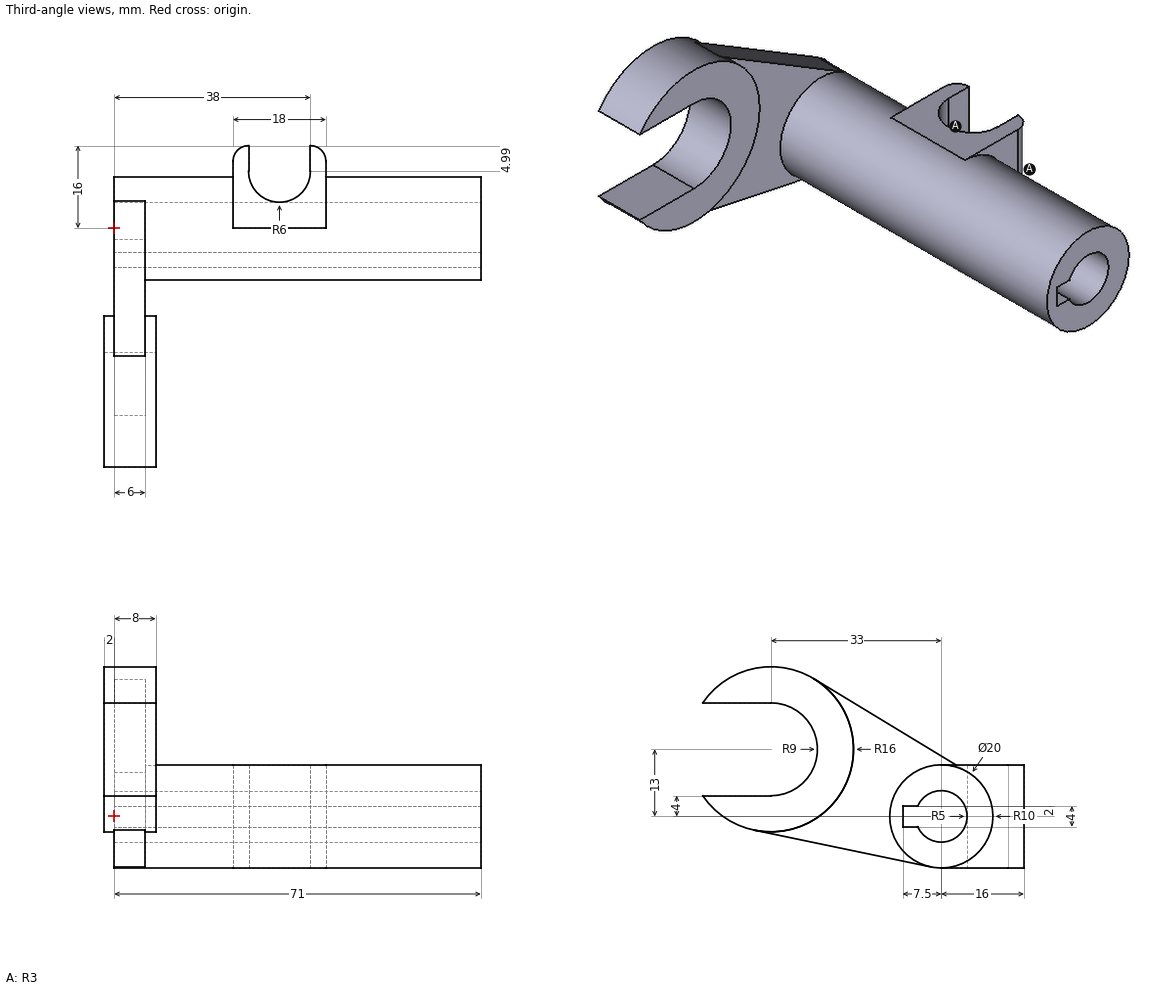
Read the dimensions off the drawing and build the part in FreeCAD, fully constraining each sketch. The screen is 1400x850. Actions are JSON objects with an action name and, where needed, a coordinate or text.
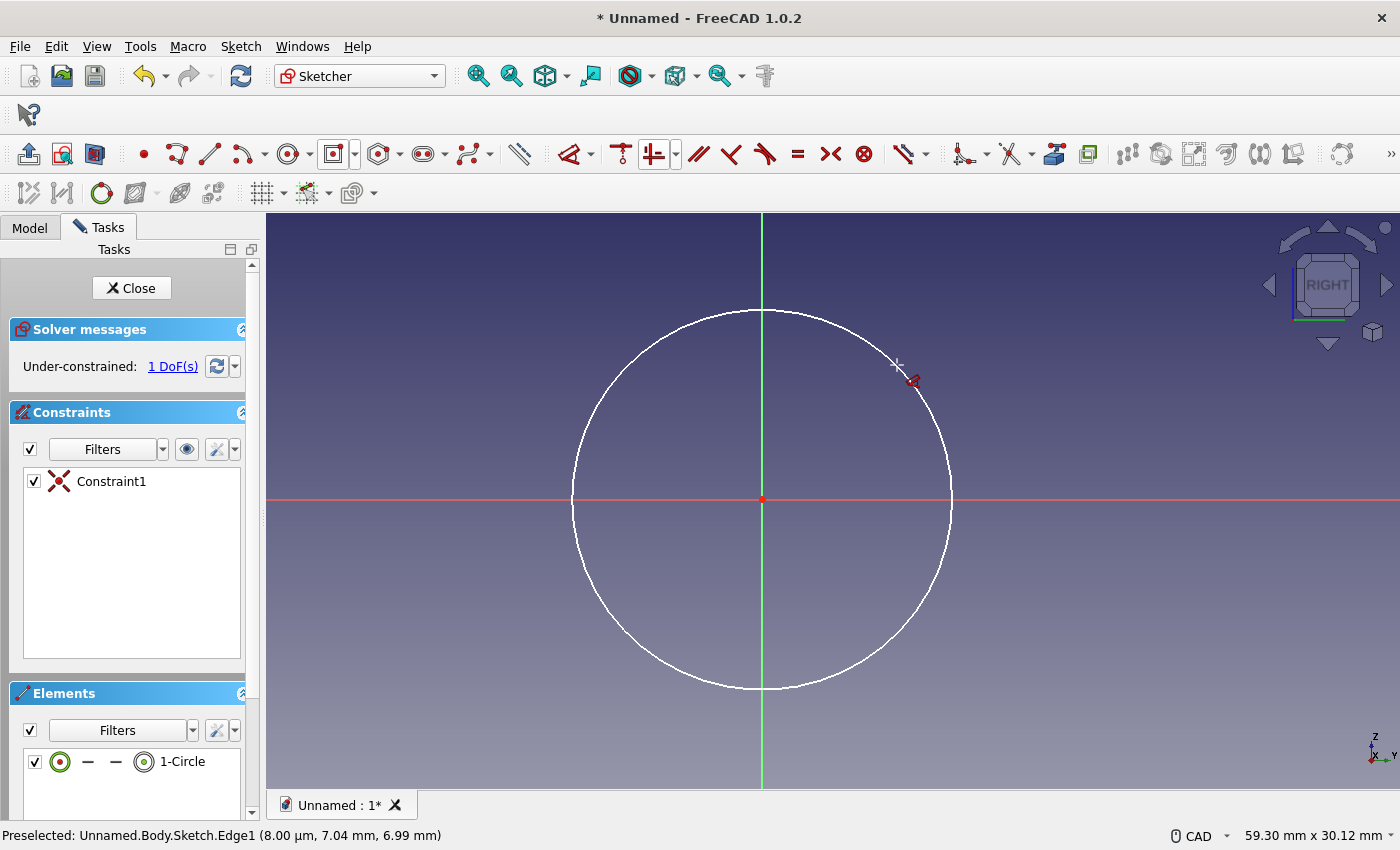
{"action": "left_click", "coordinate": [896, 365]}
{"action": "left_click", "coordinate": [919, 342]}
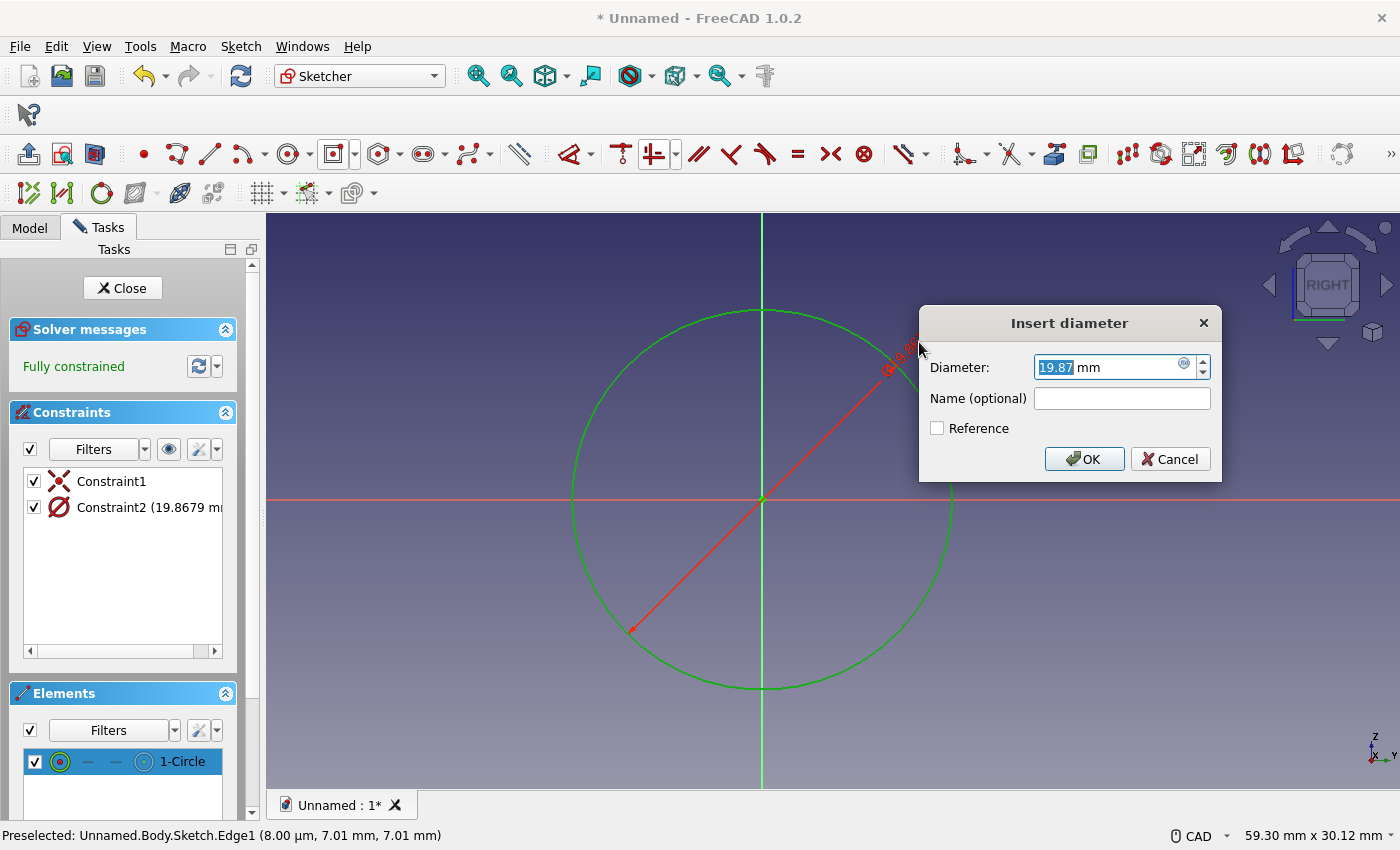
{"action": "type", "text": "20"}
{"action": "key", "text": "Return"}
{"action": "key", "text": "Escape"}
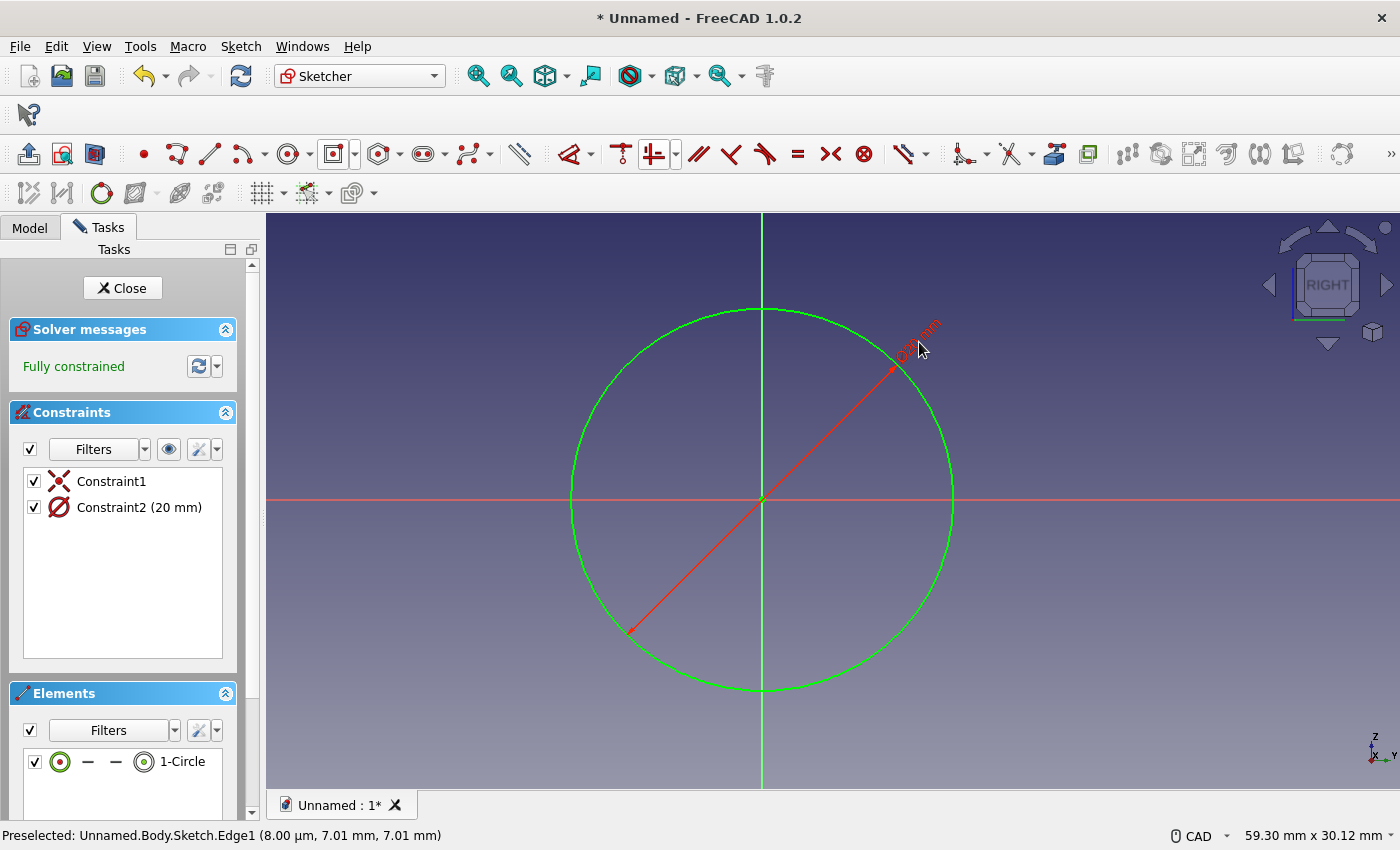
{"action": "left_click", "coordinate": [123, 288]}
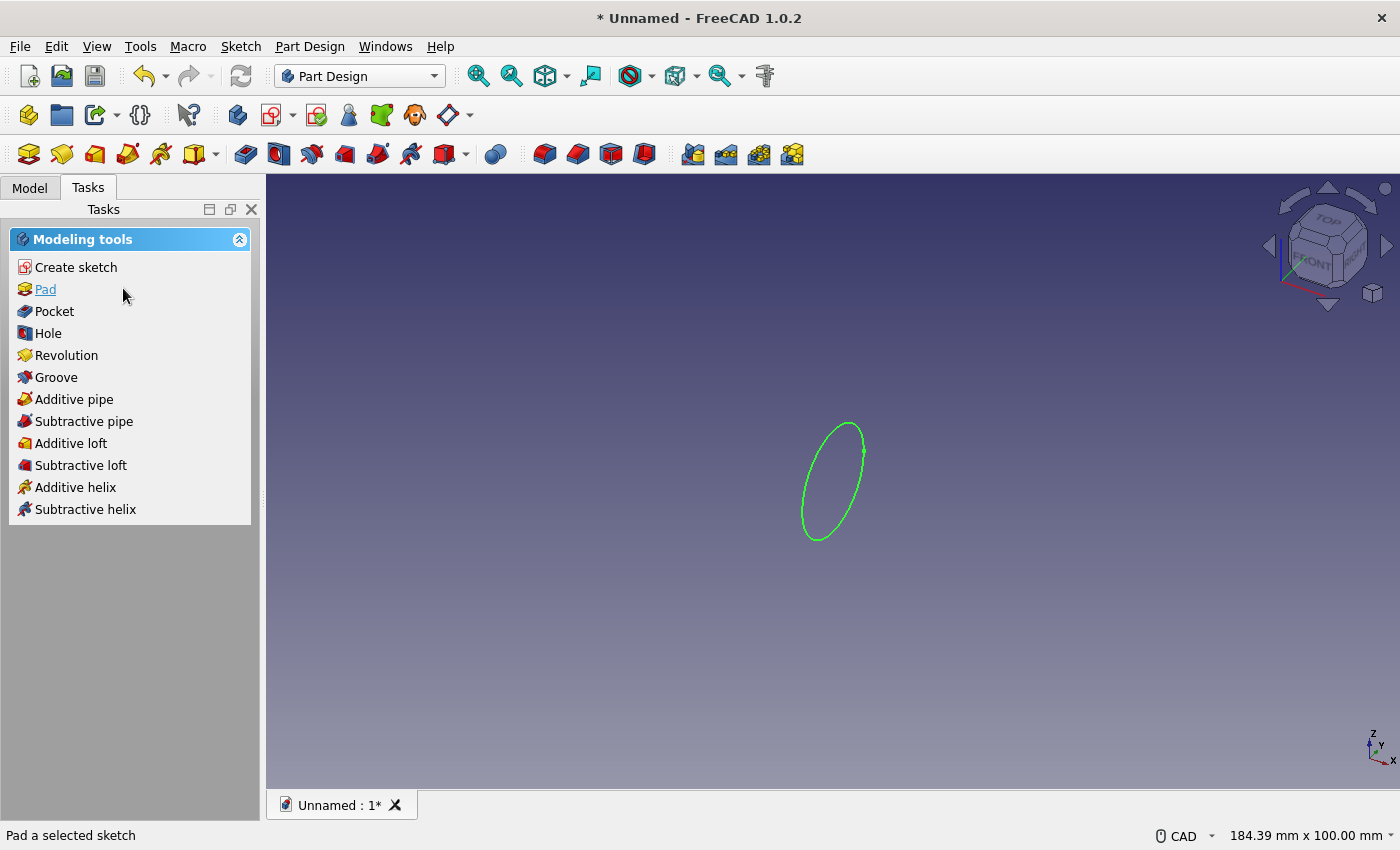
{"action": "left_click", "coordinate": [29, 154]}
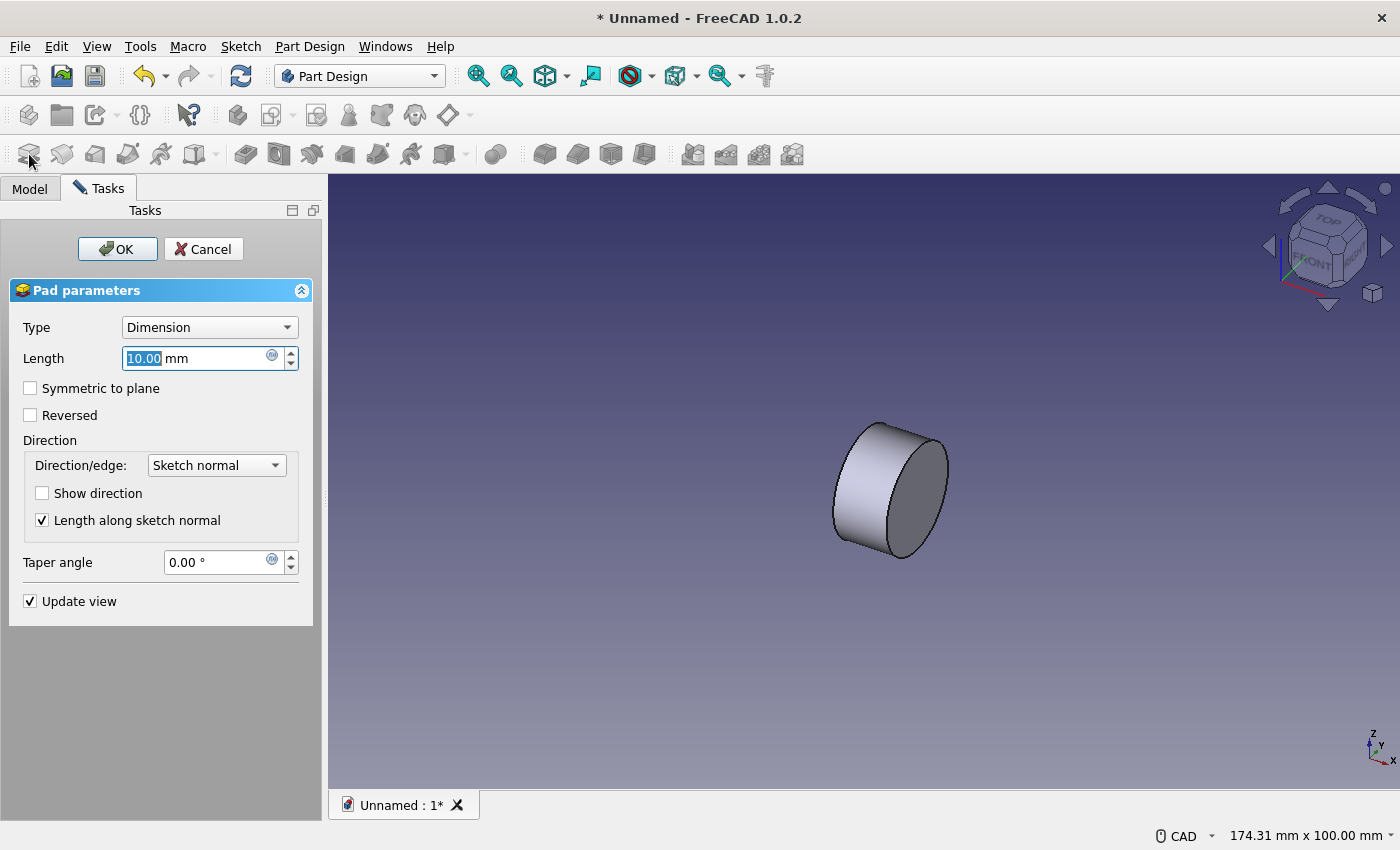
{"action": "type", "text": "71"}
{"action": "key", "text": "Tab"}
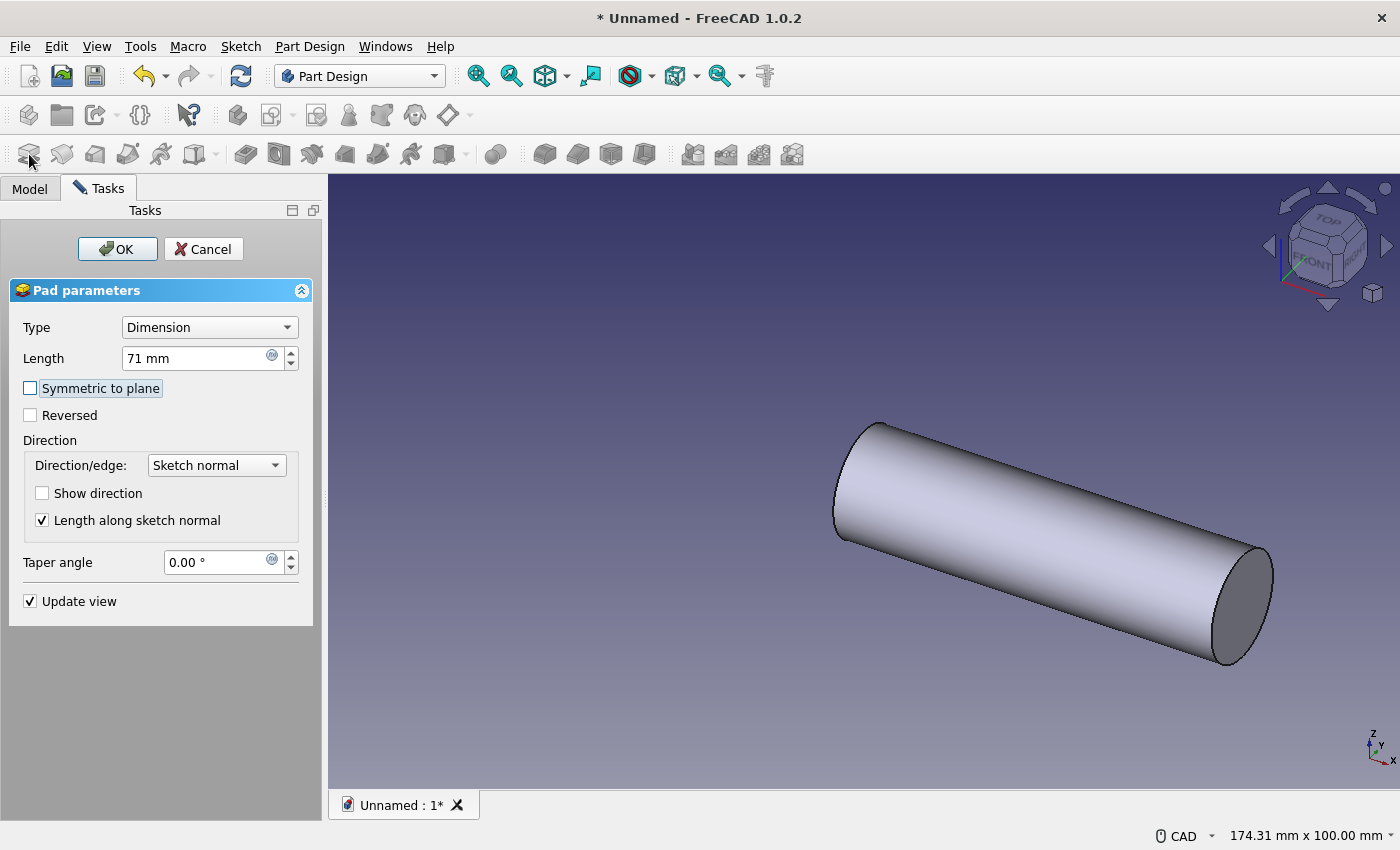
{"action": "left_click", "coordinate": [118, 249]}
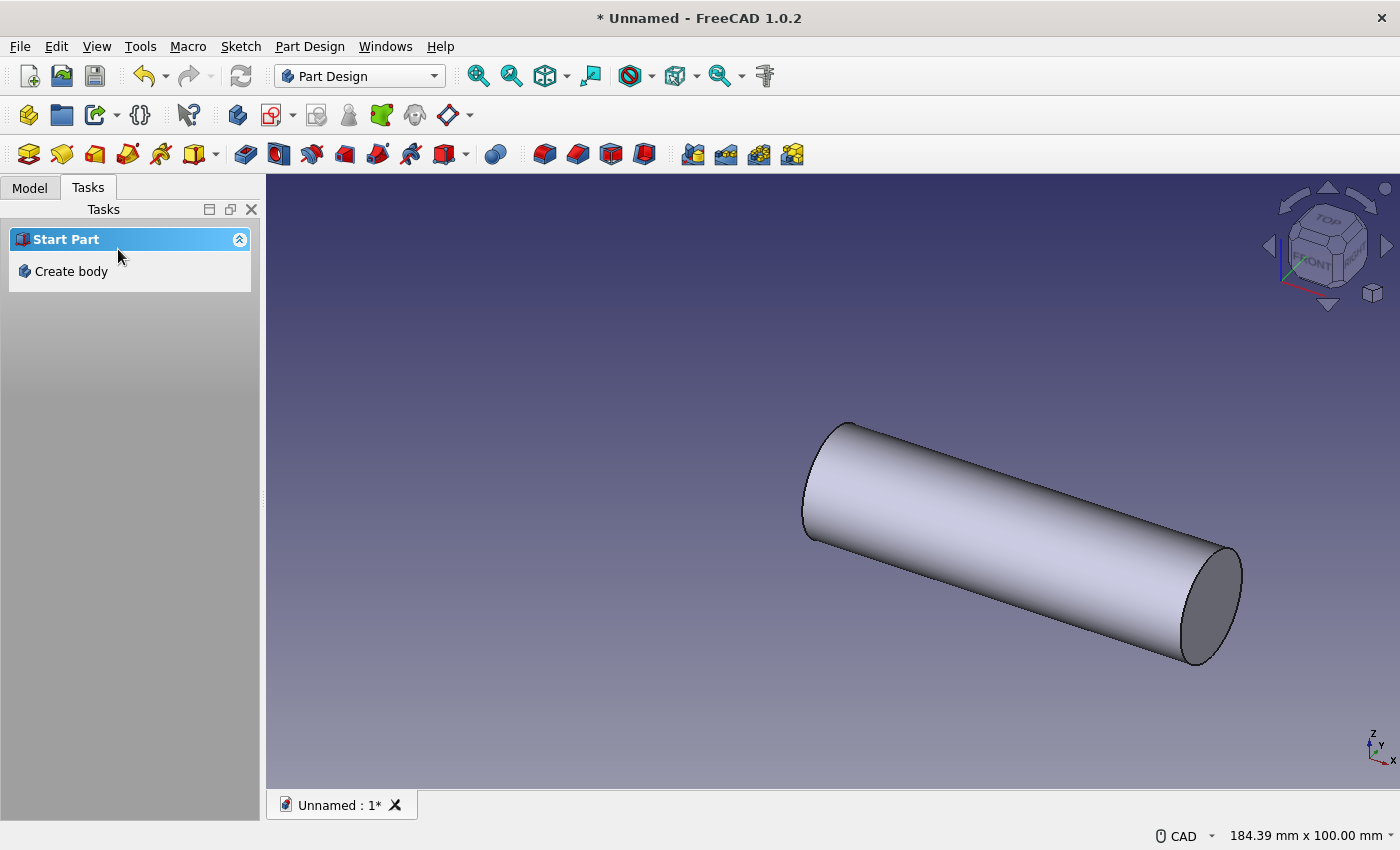
{"action": "left_click", "coordinate": [1211, 606]}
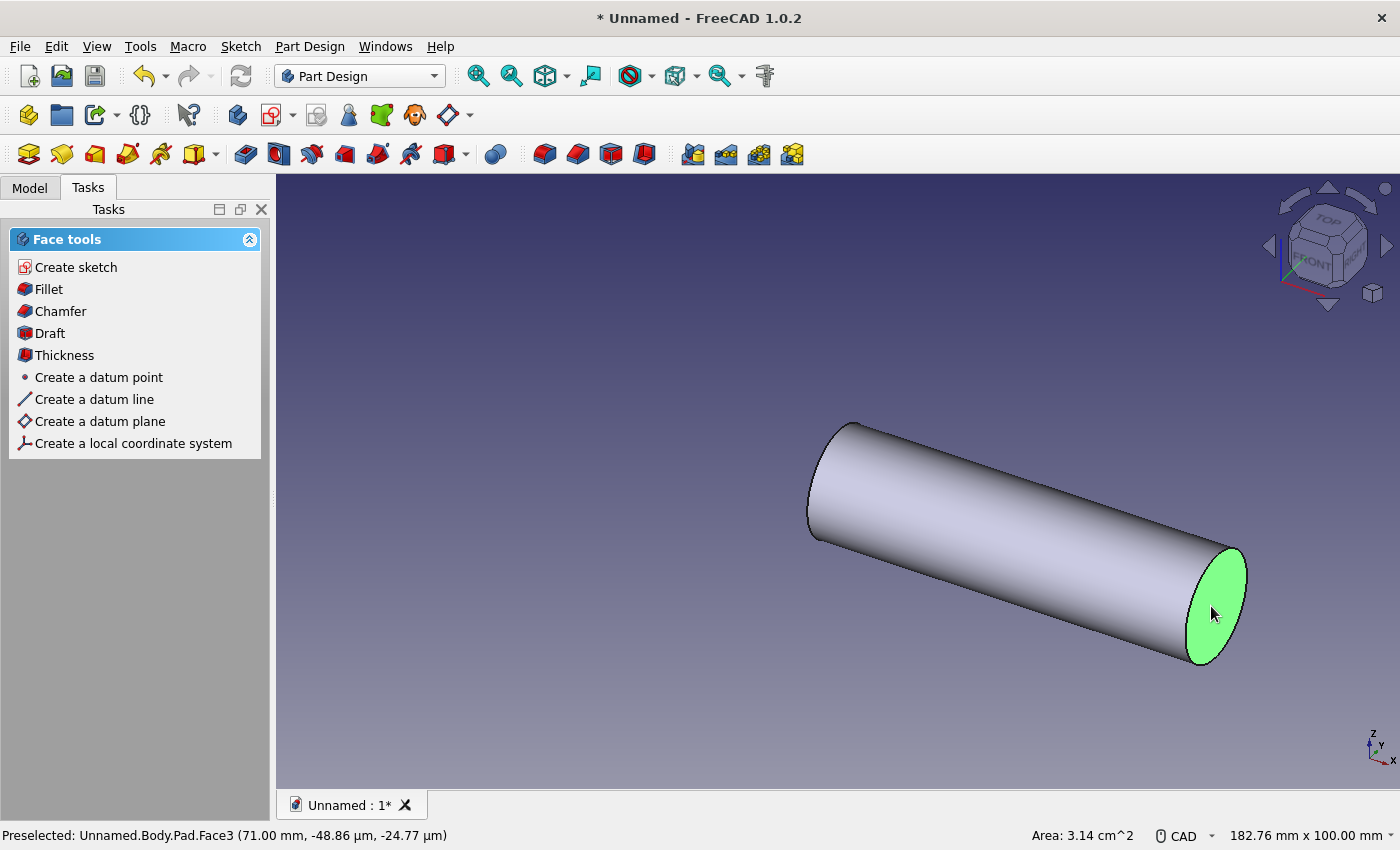
{"action": "left_click", "coordinate": [270, 116]}